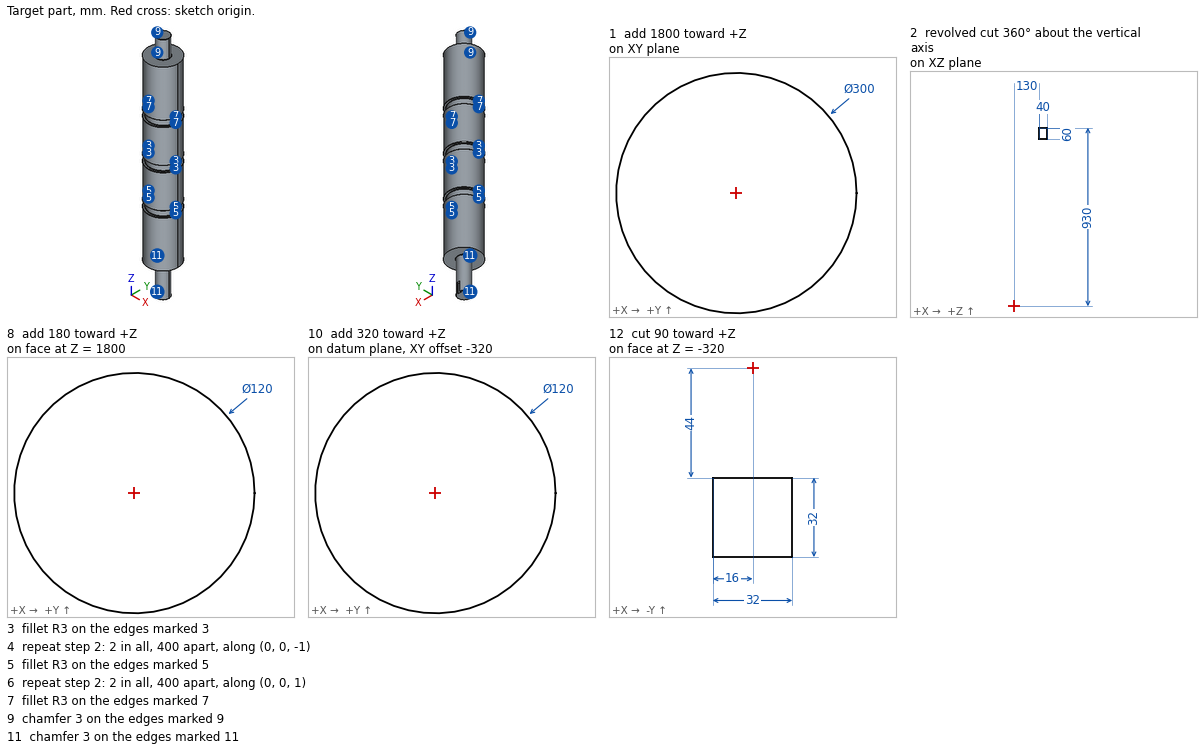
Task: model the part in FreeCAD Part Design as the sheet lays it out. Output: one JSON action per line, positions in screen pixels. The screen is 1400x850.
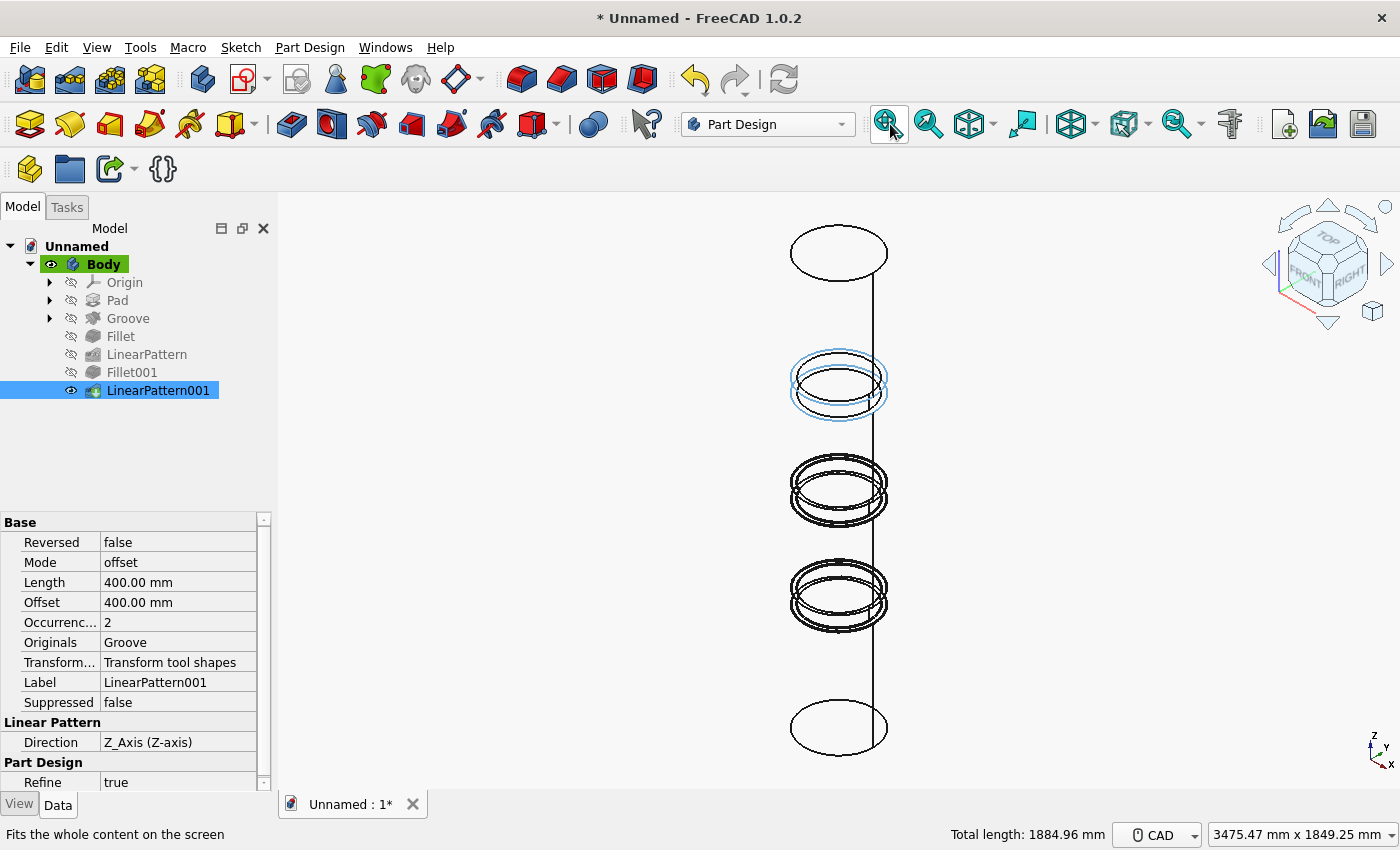
{"action": "left_click", "coordinate": [809, 359], "text": "ctrl"}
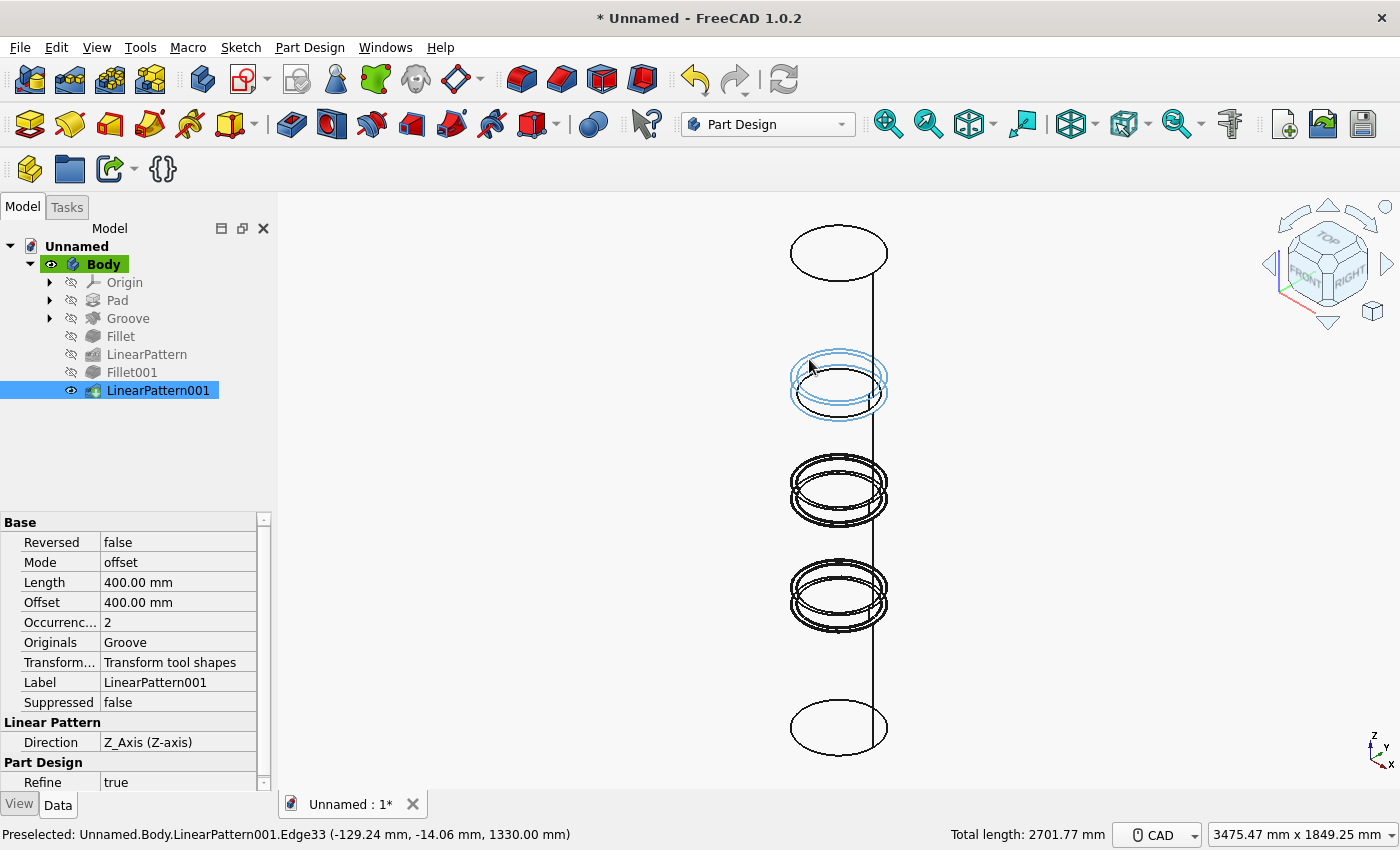
{"action": "left_click", "coordinate": [809, 375], "text": "ctrl"}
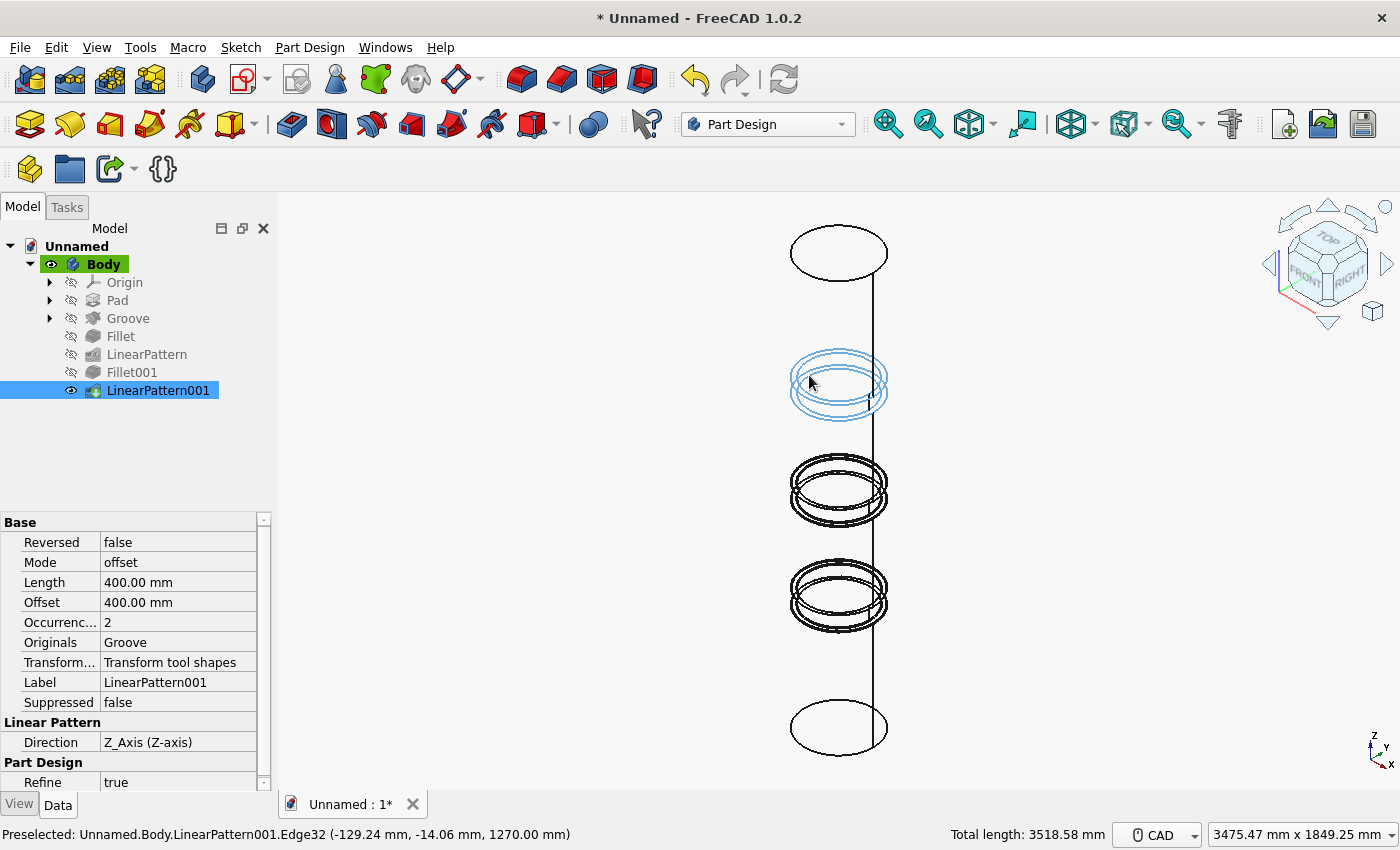
{"action": "key", "text": "v 1"}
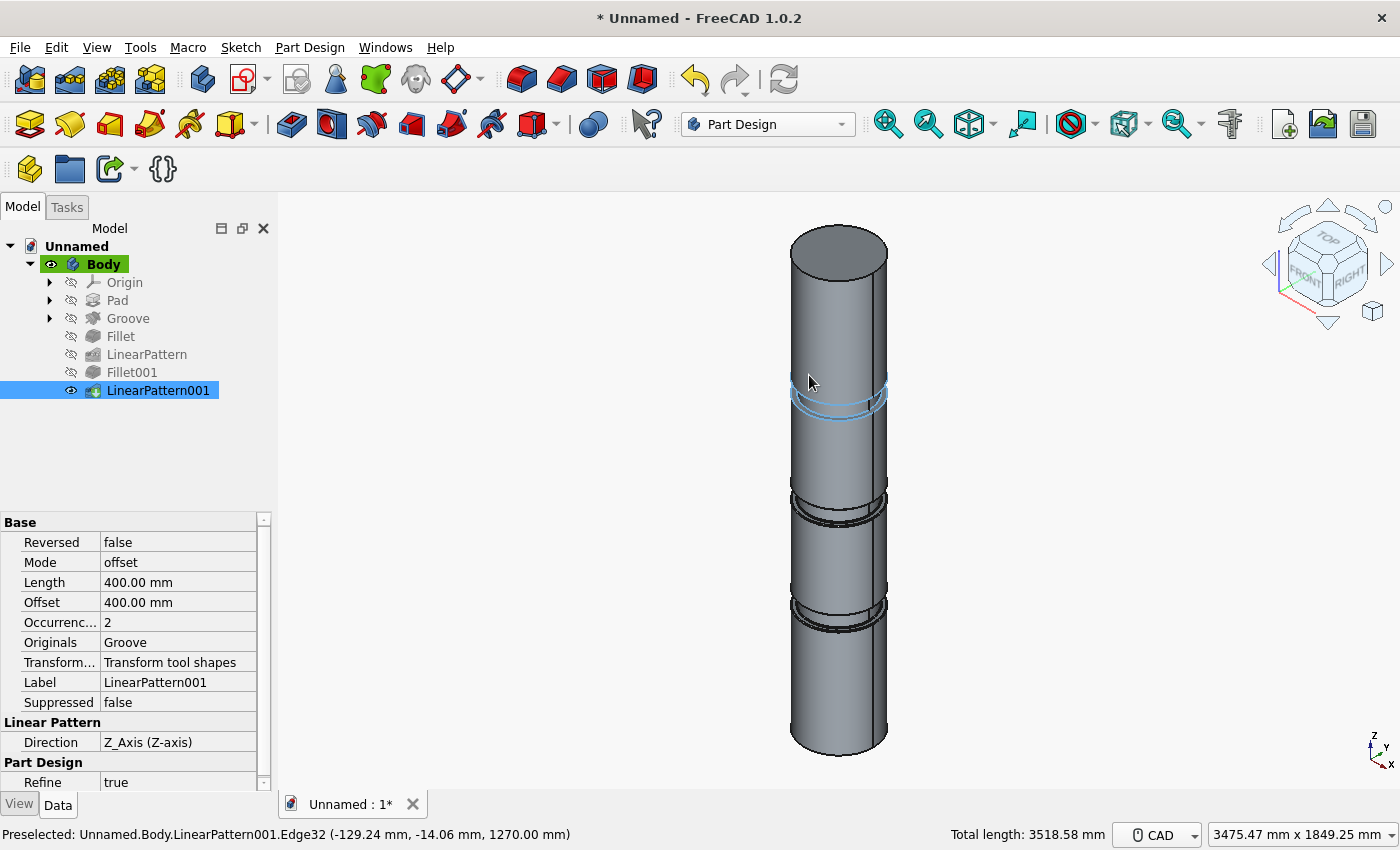
{"action": "left_click", "coordinate": [522, 80]}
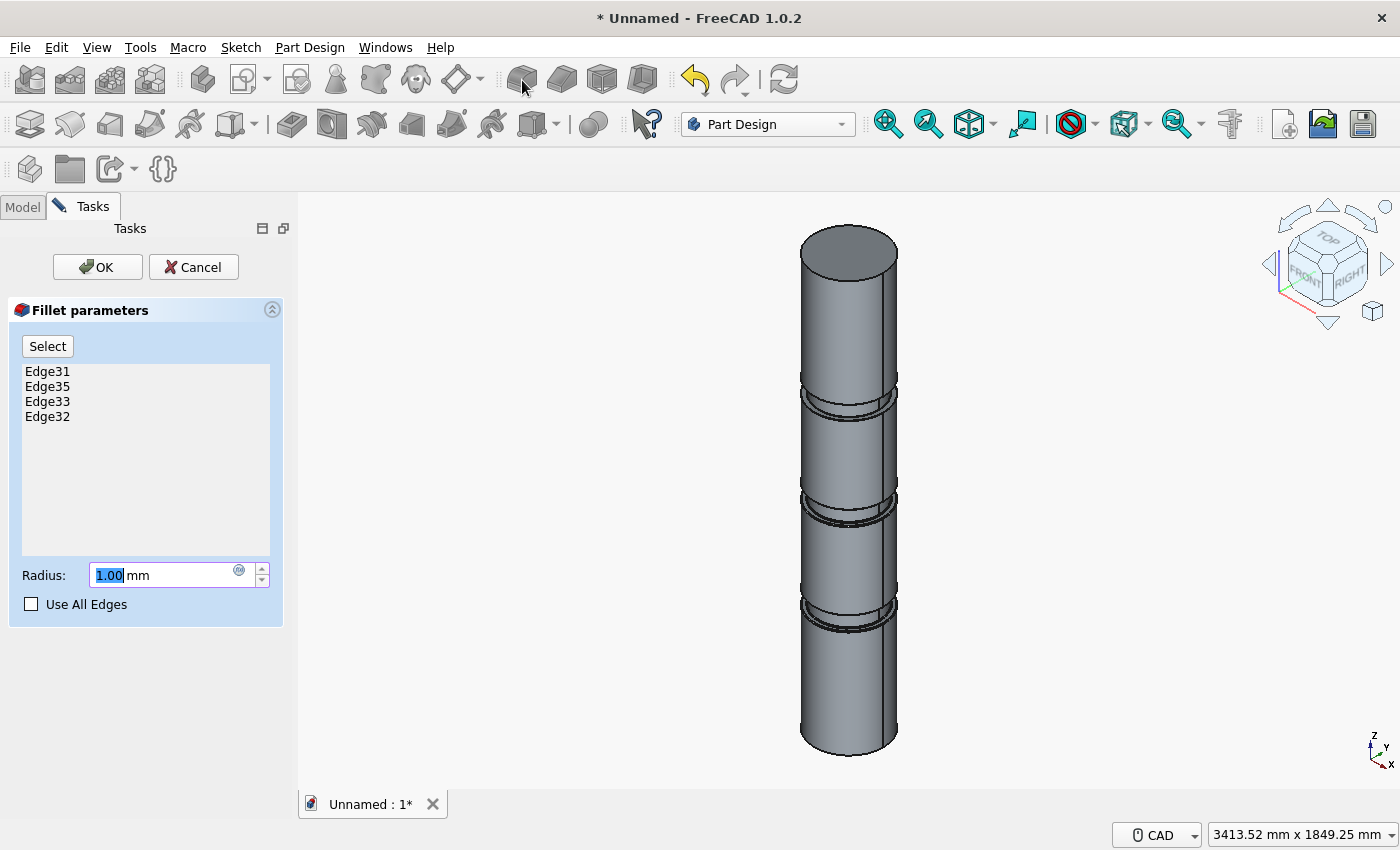
{"action": "type", "text": "3"}
{"action": "key", "text": "Tab"}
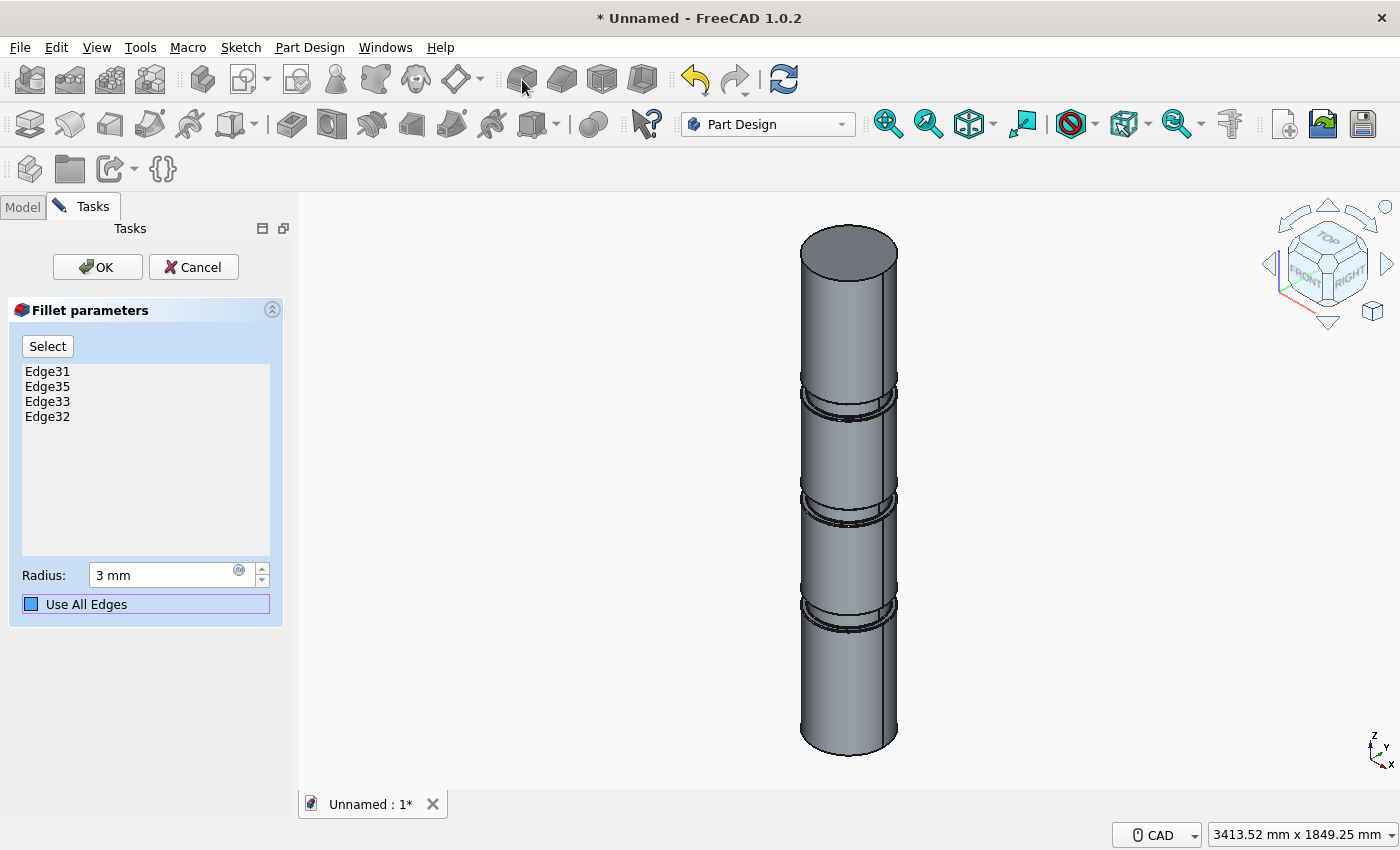
{"action": "left_click", "coordinate": [98, 267]}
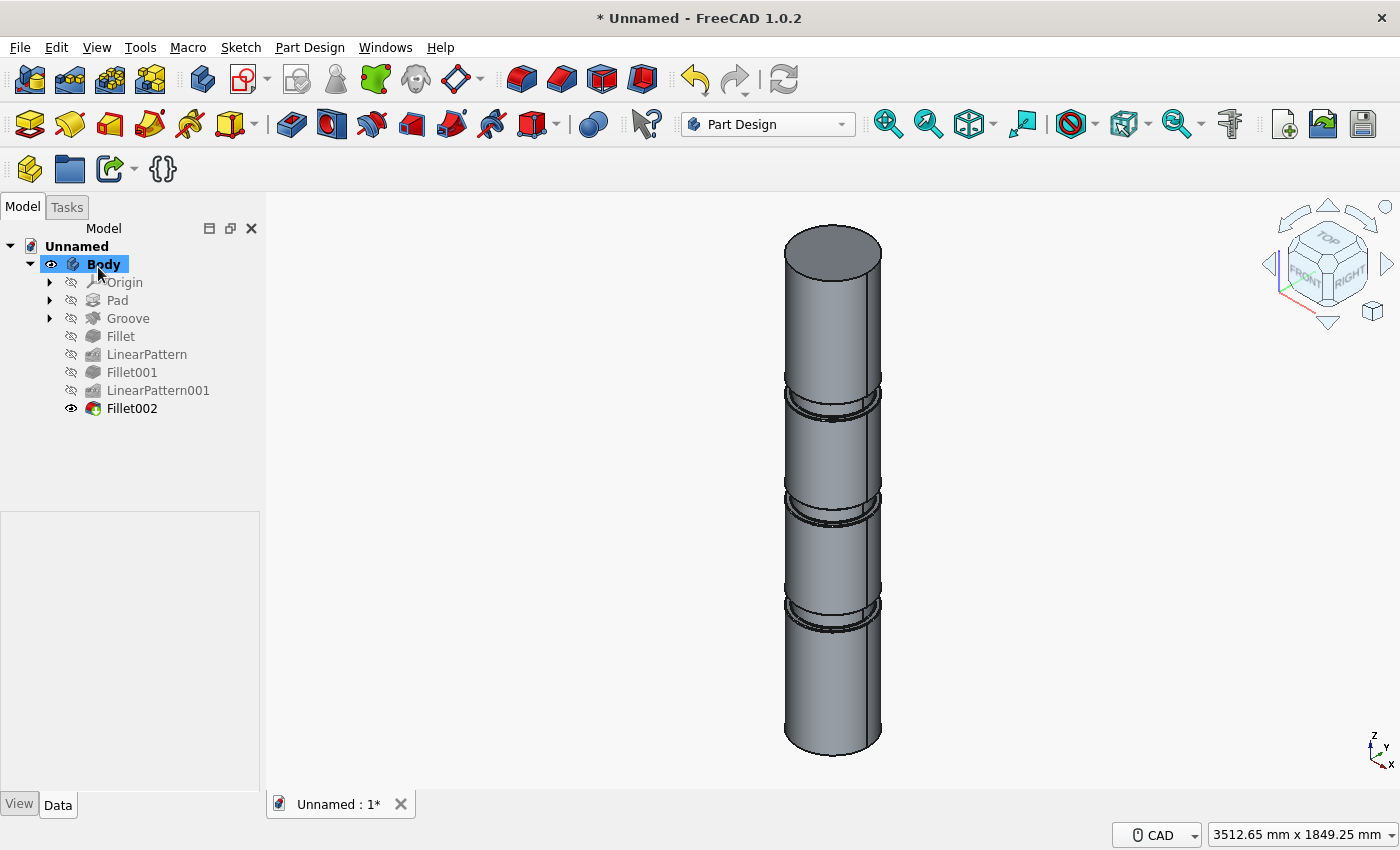
{"action": "left_click", "coordinate": [833, 252]}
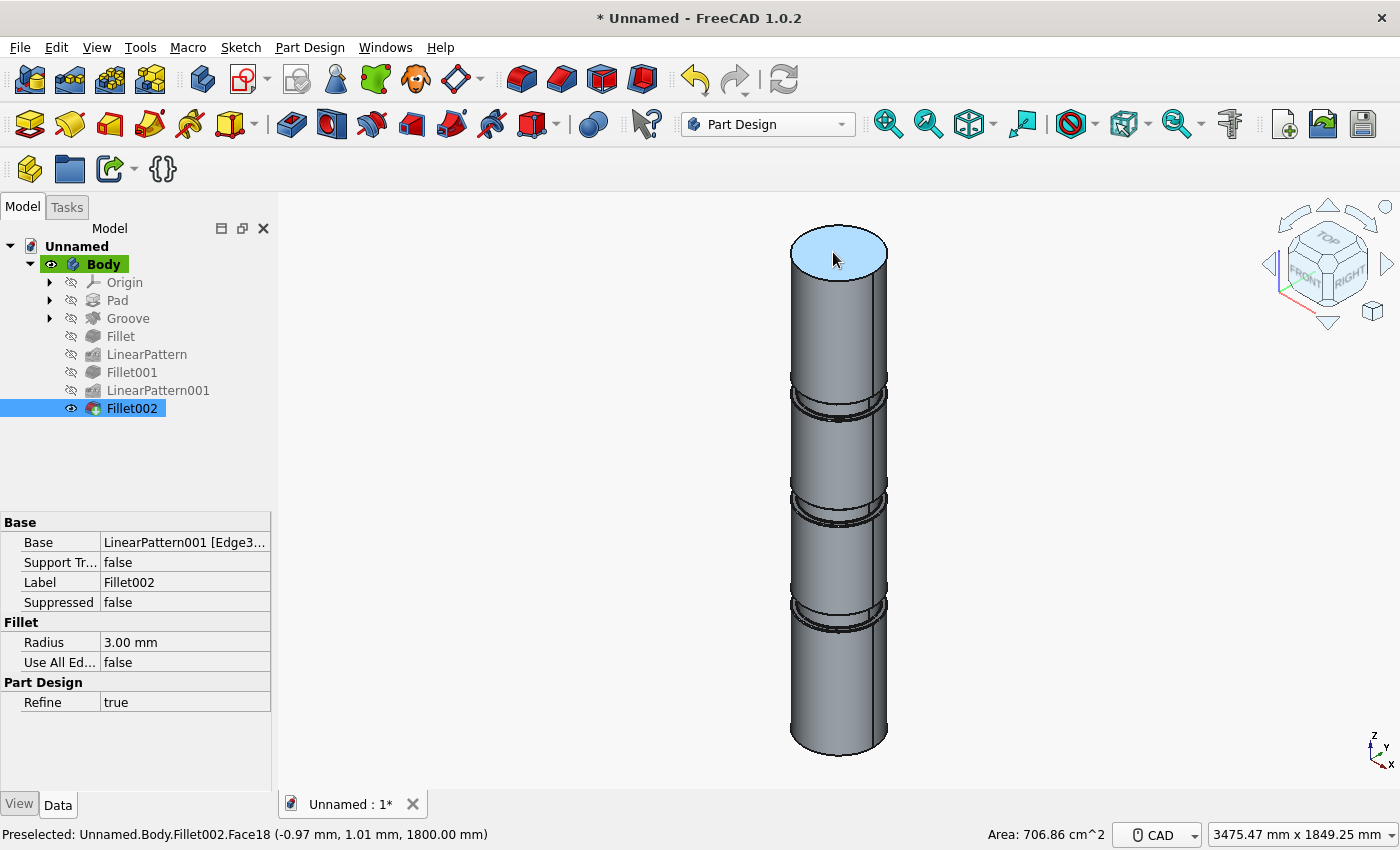
{"action": "left_click", "coordinate": [244, 80]}